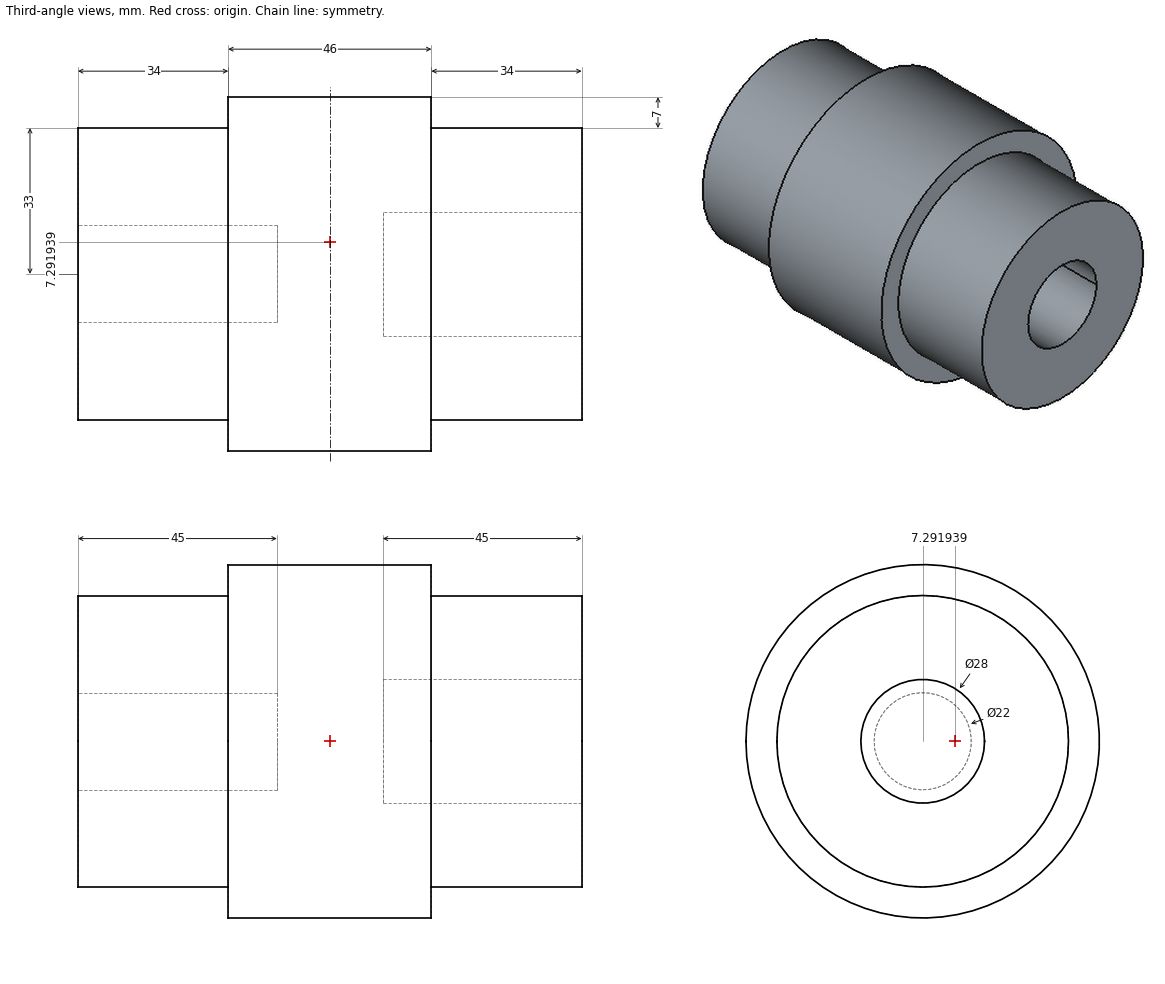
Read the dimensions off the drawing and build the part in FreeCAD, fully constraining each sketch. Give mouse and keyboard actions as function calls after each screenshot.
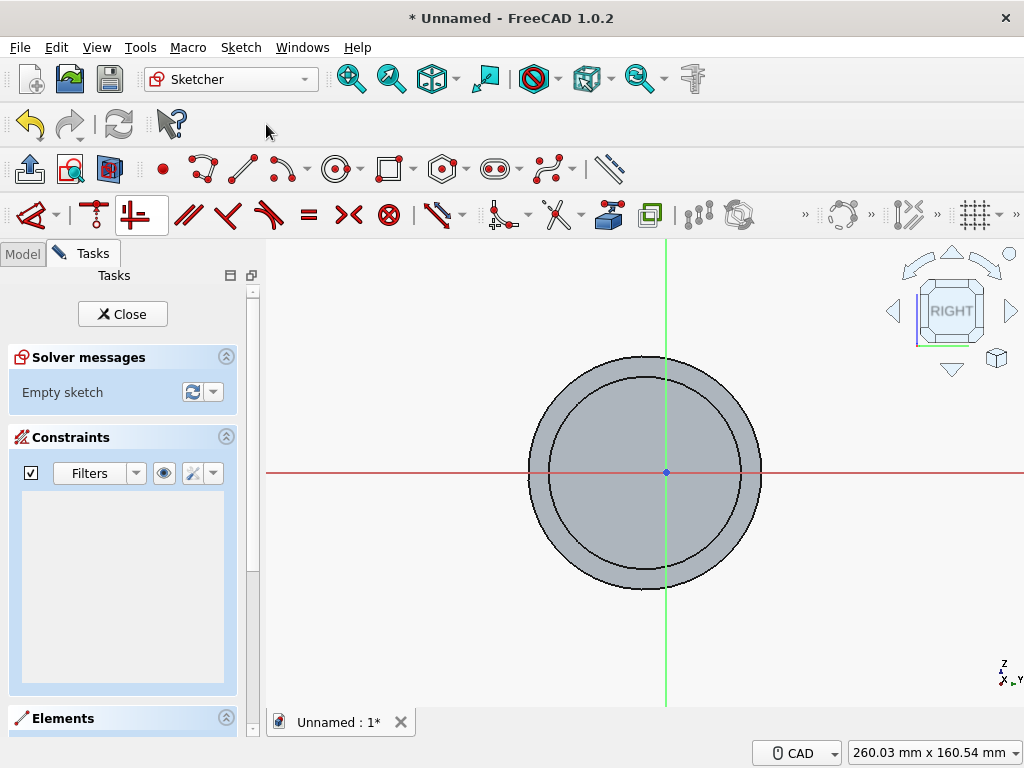
scroll(674, 473, up, 6)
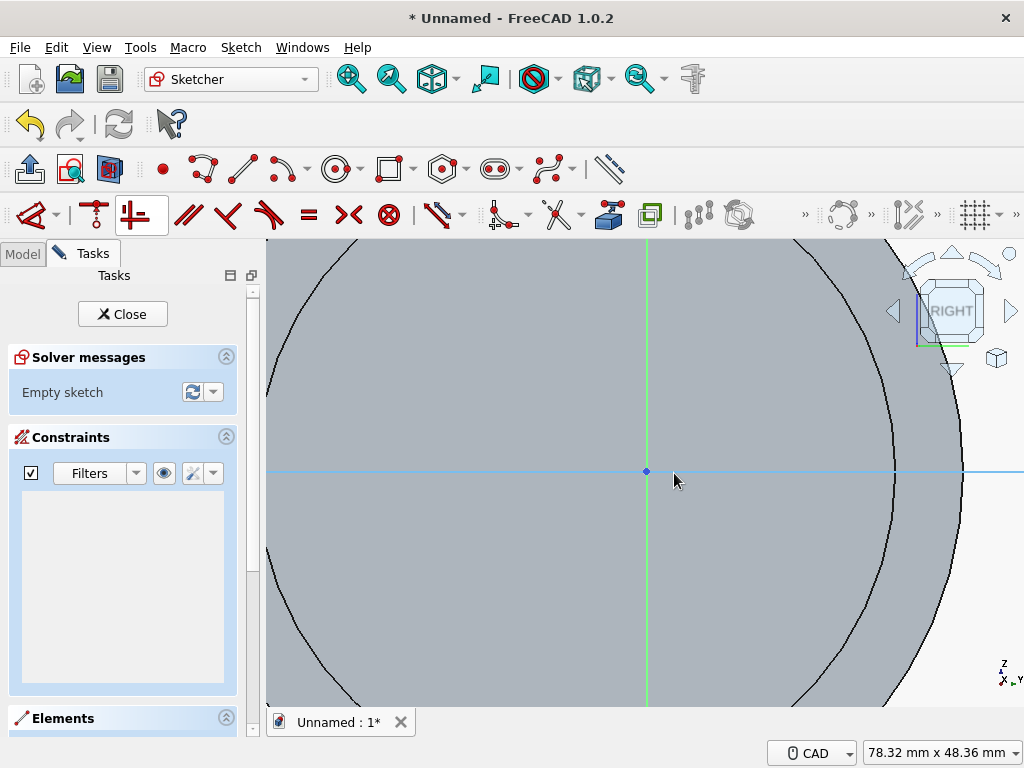
click(336, 170)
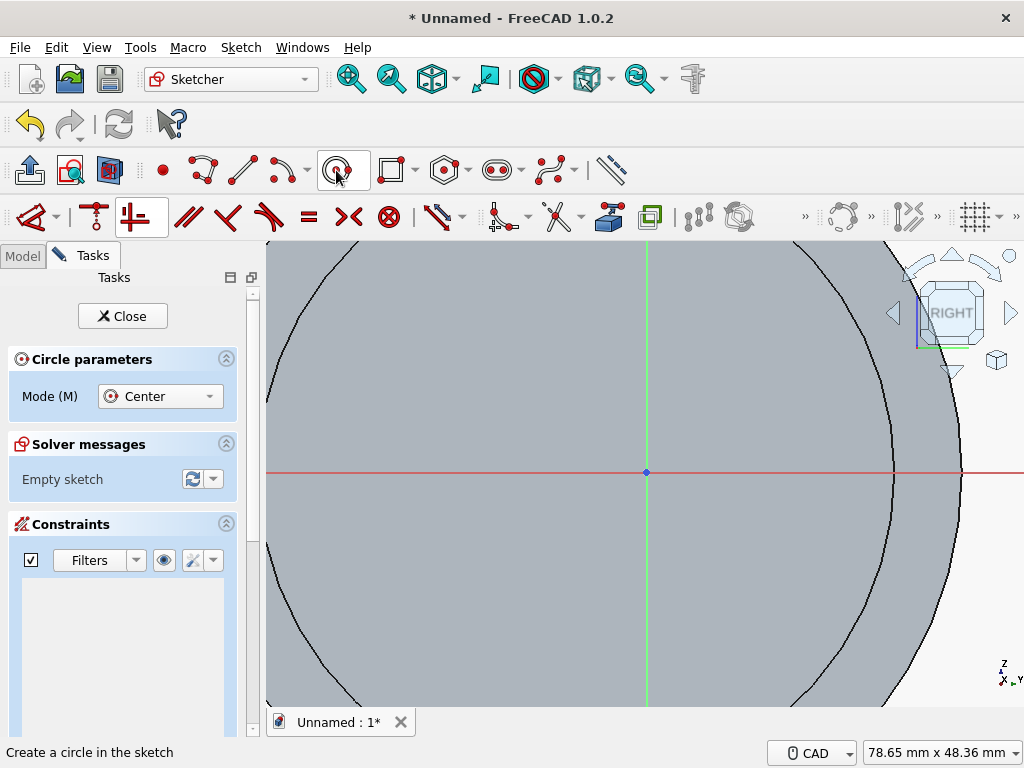
click(576, 473)
move(672, 377)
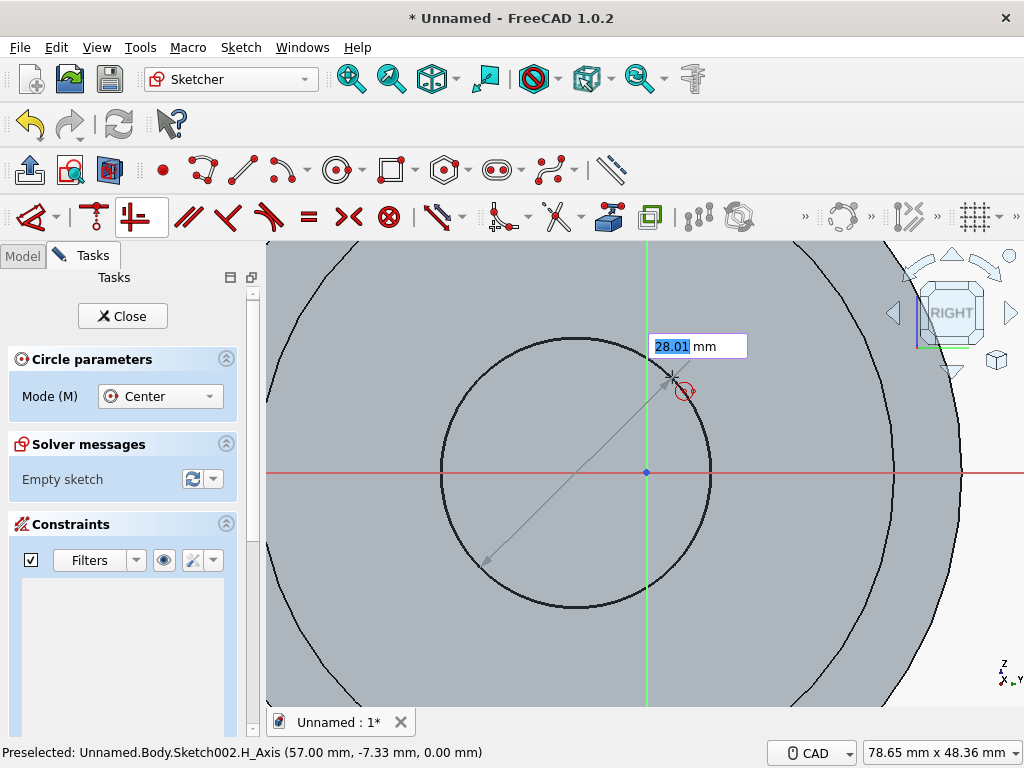
text(28)
key(Return)
key(Escape)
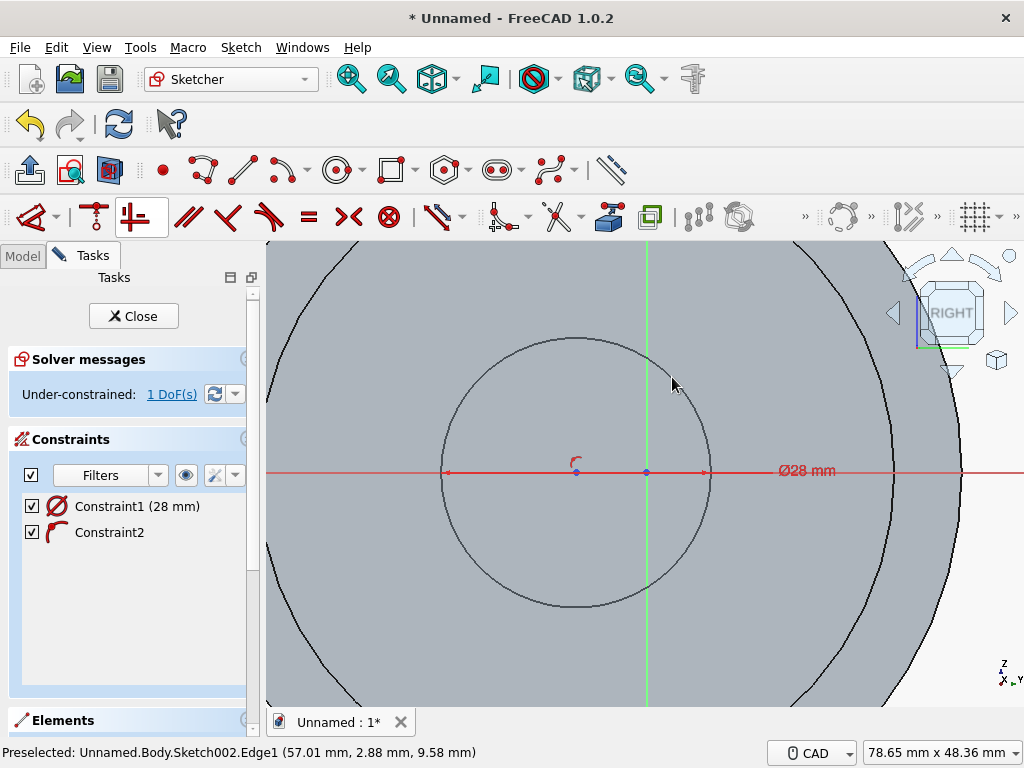
click(32, 218)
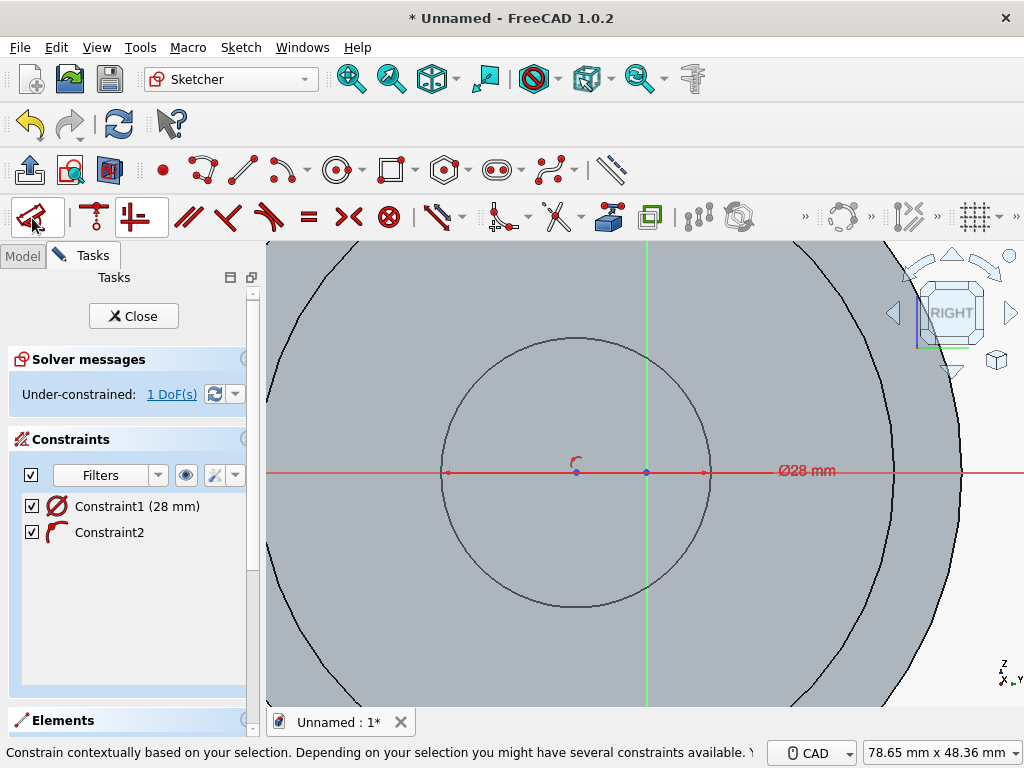
click(576, 473)
click(611, 507)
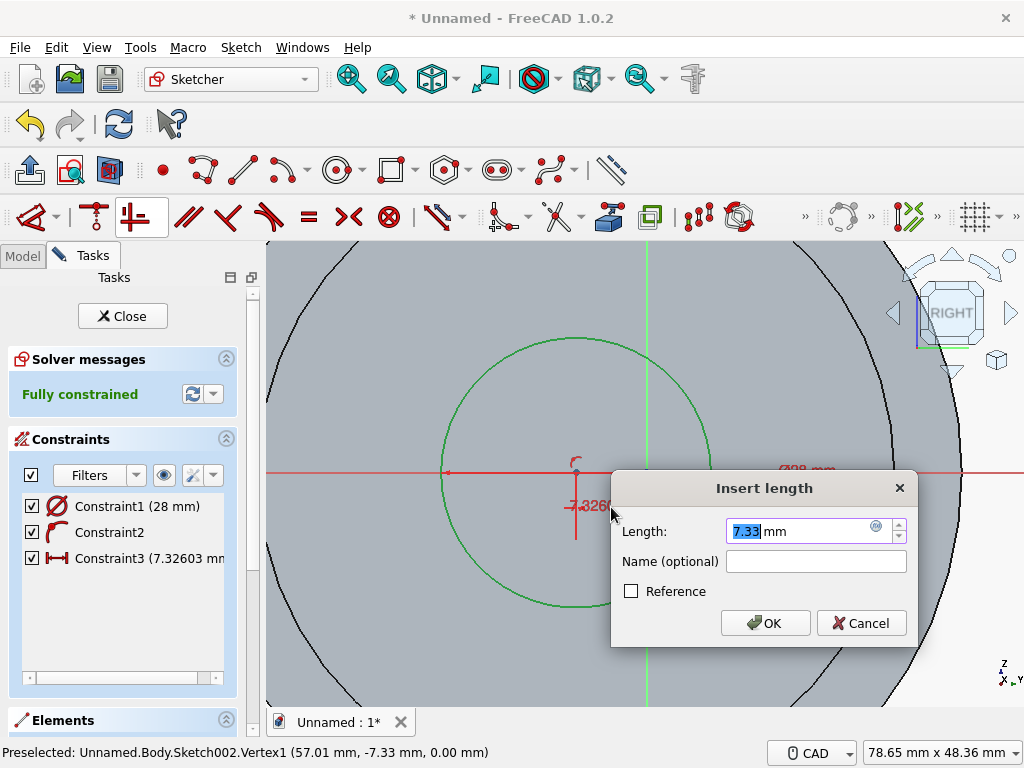
text(7.291939)
key(Return)
key(Escape)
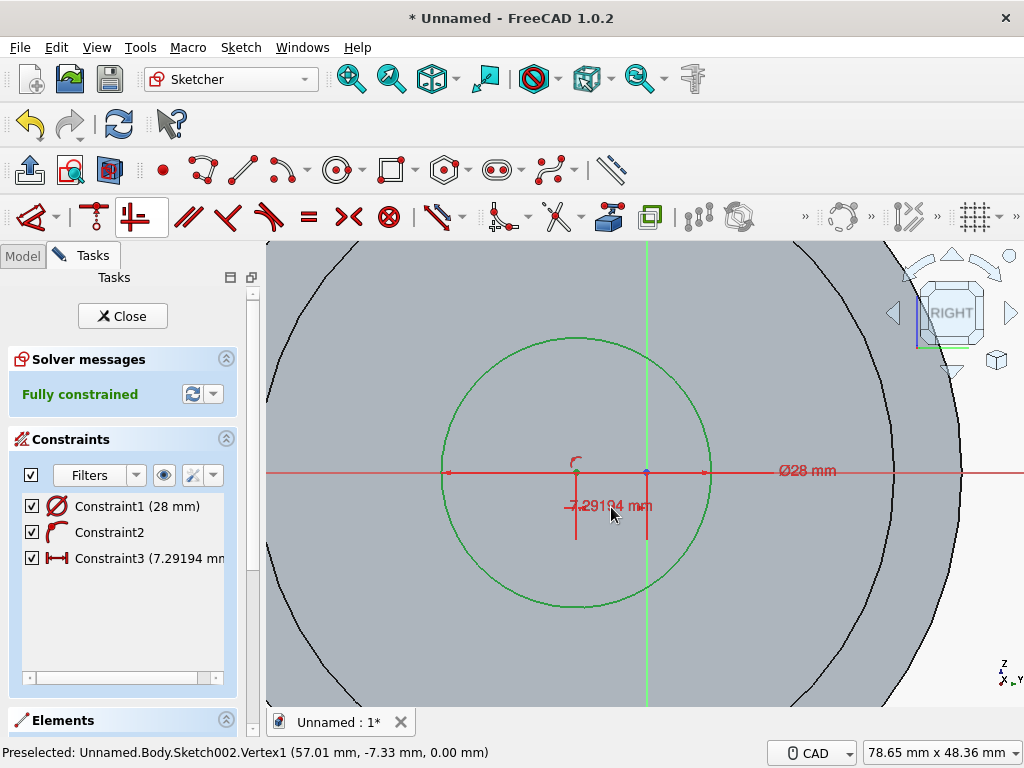
click(123, 316)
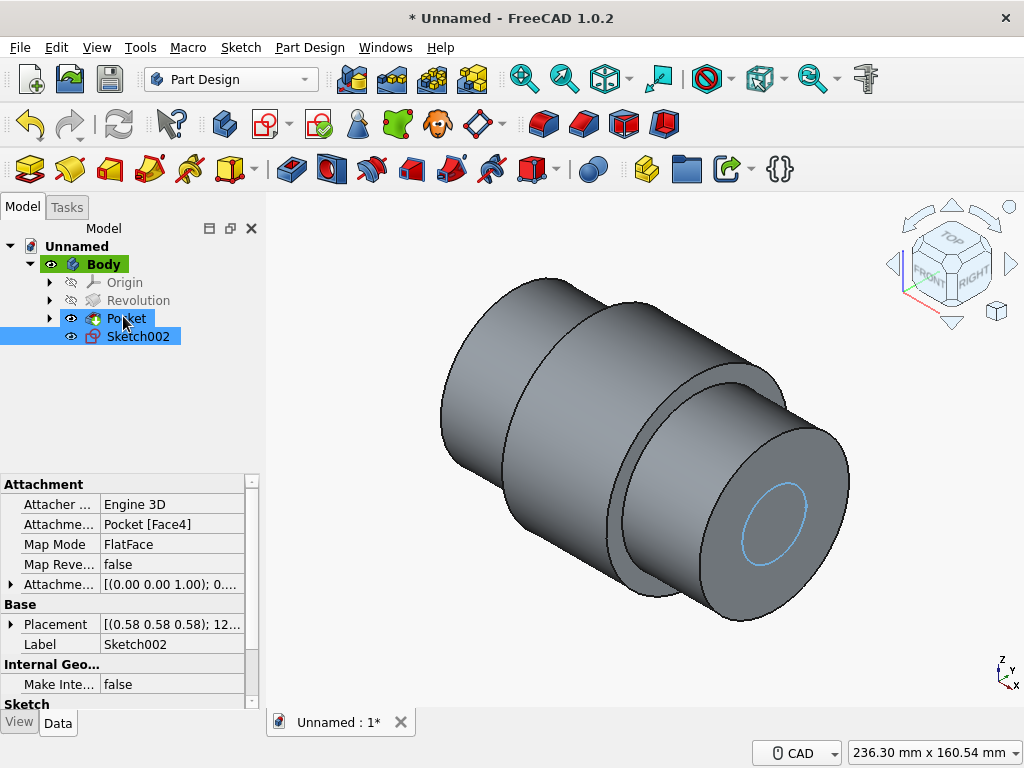
click(292, 170)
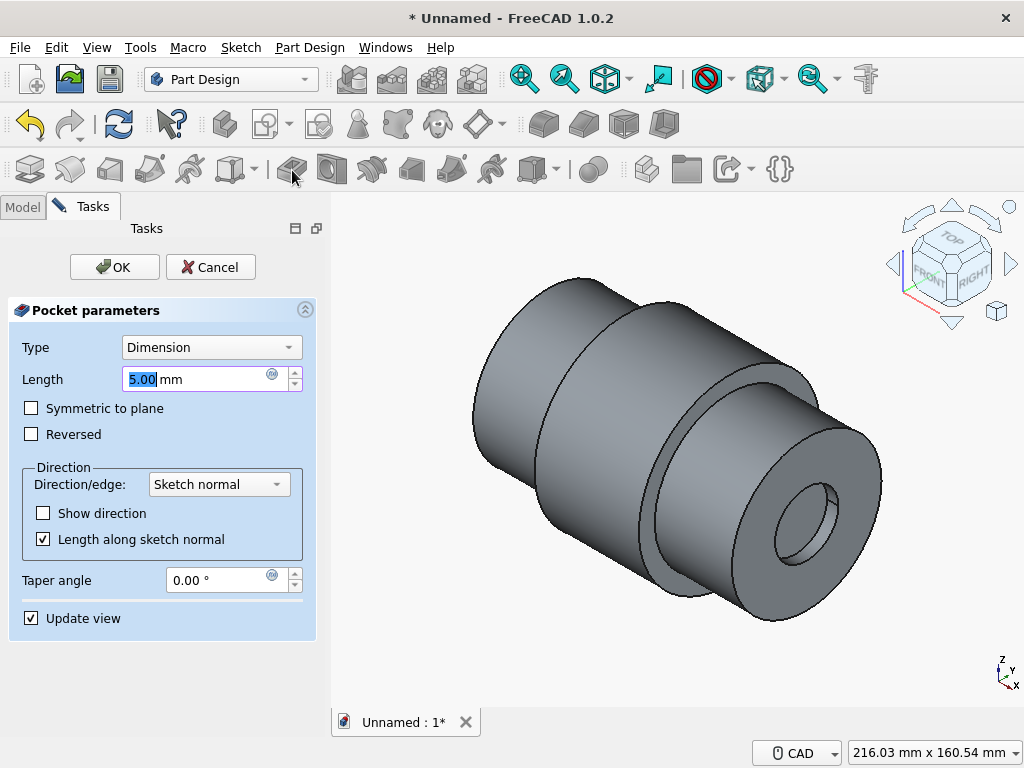
text(45)
key(Tab)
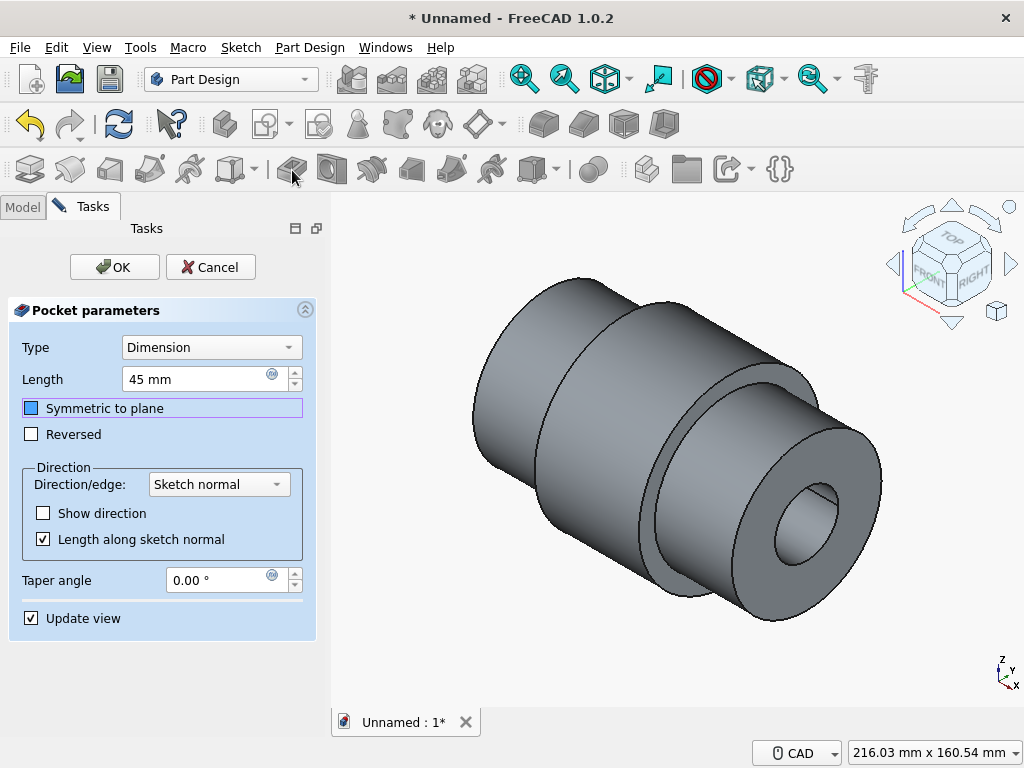
click(115, 267)